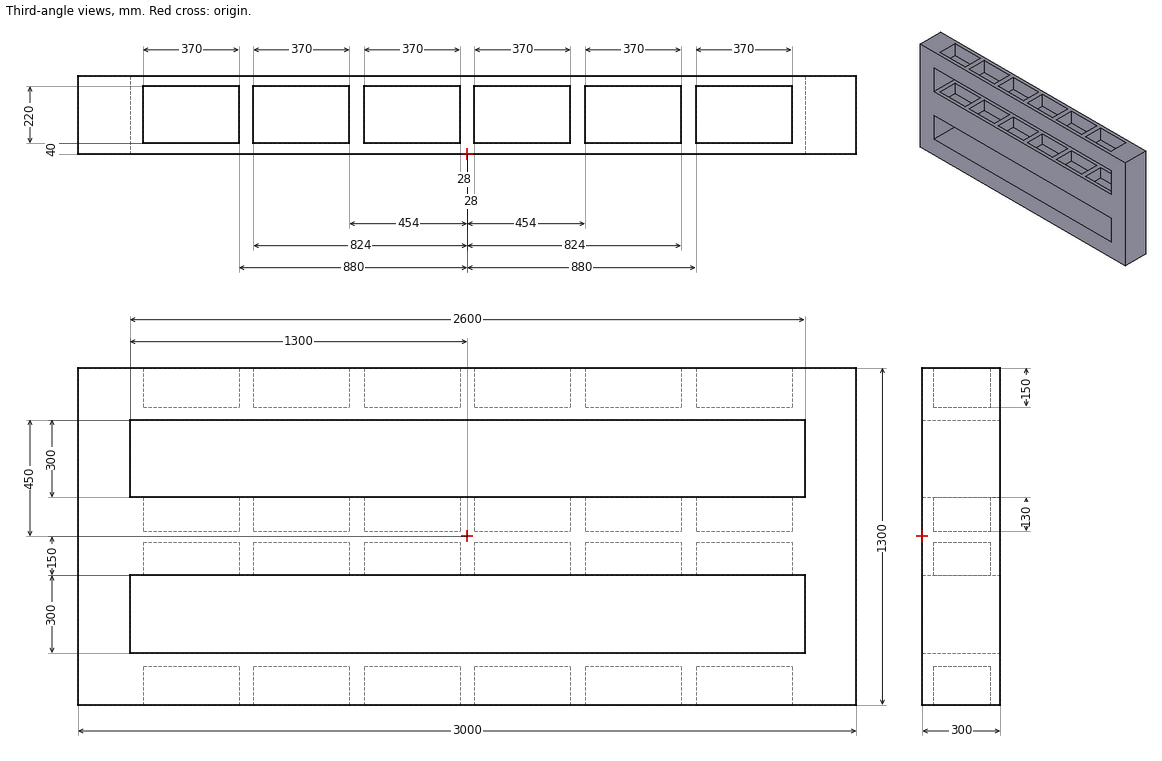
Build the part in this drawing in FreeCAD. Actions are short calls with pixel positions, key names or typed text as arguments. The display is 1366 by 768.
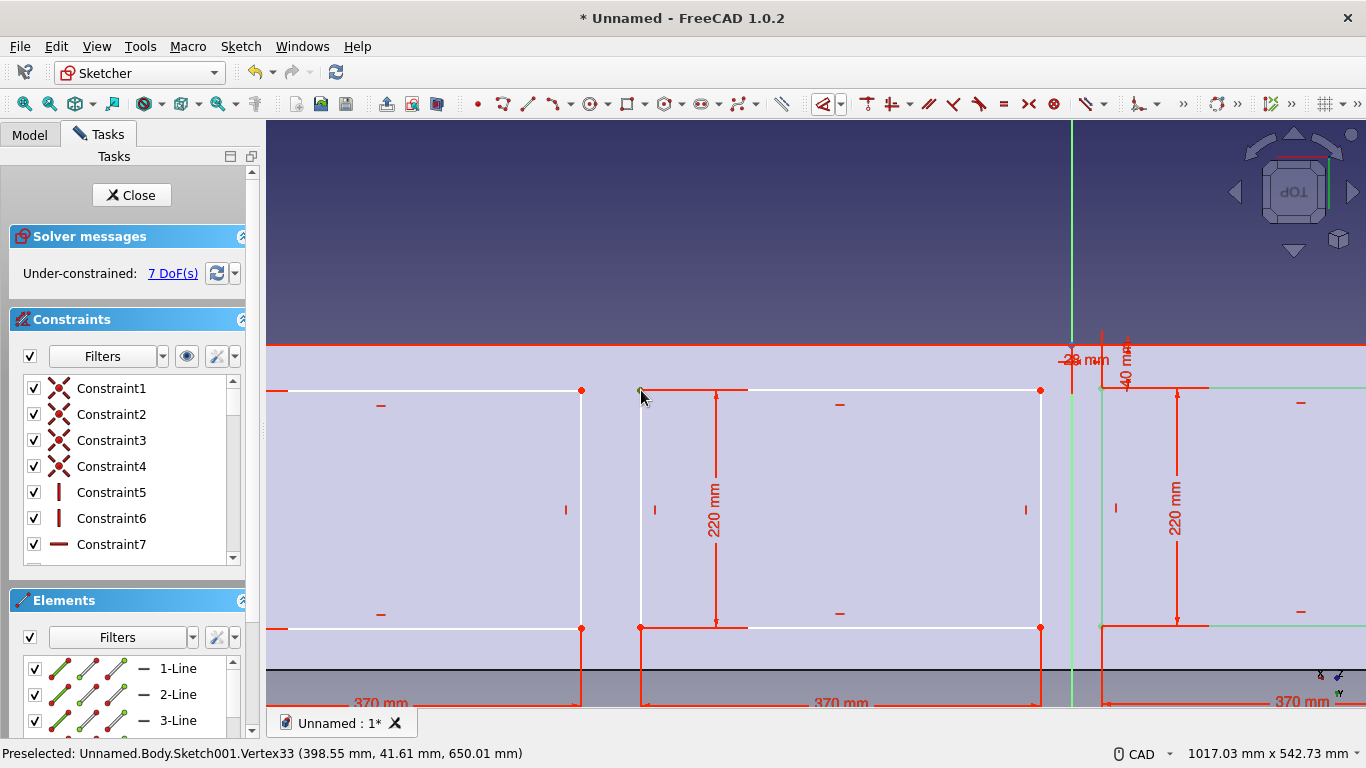
key(i)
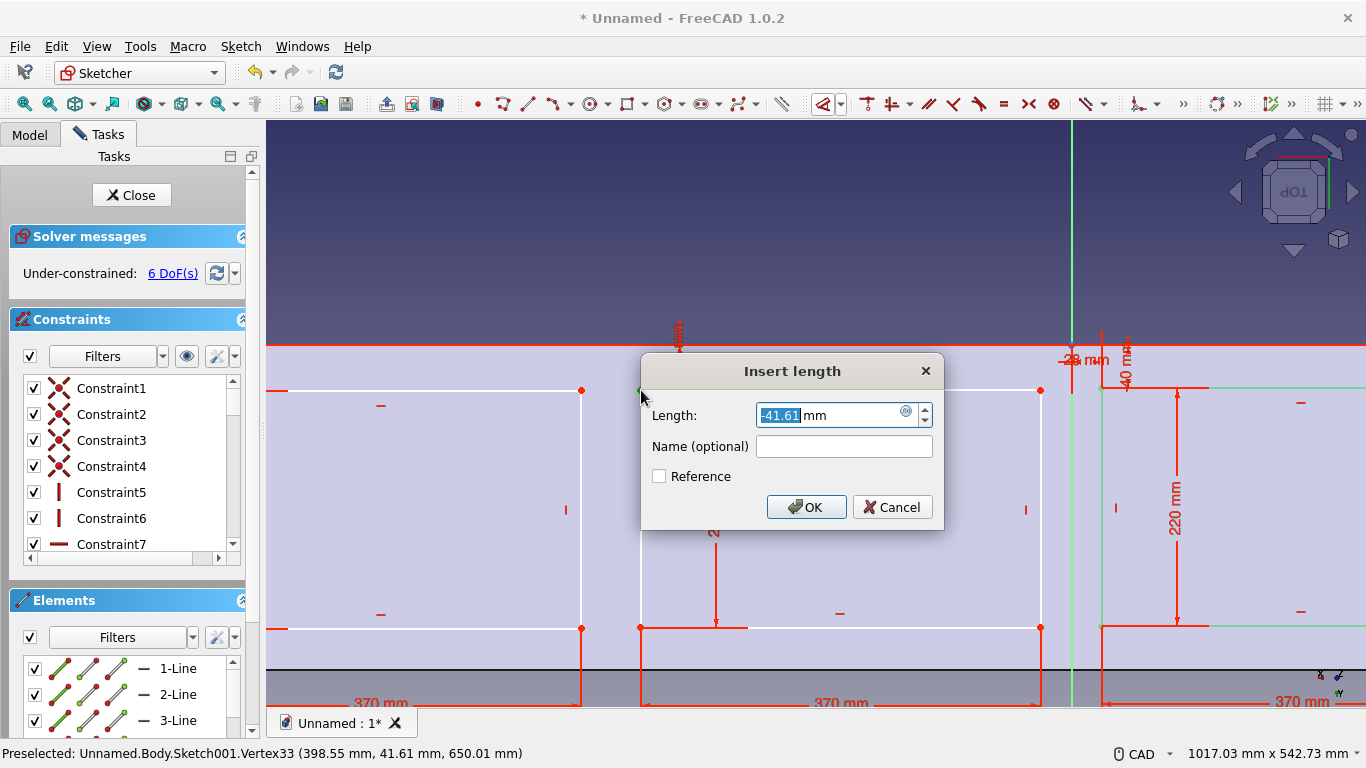
text(-40)
key(Return)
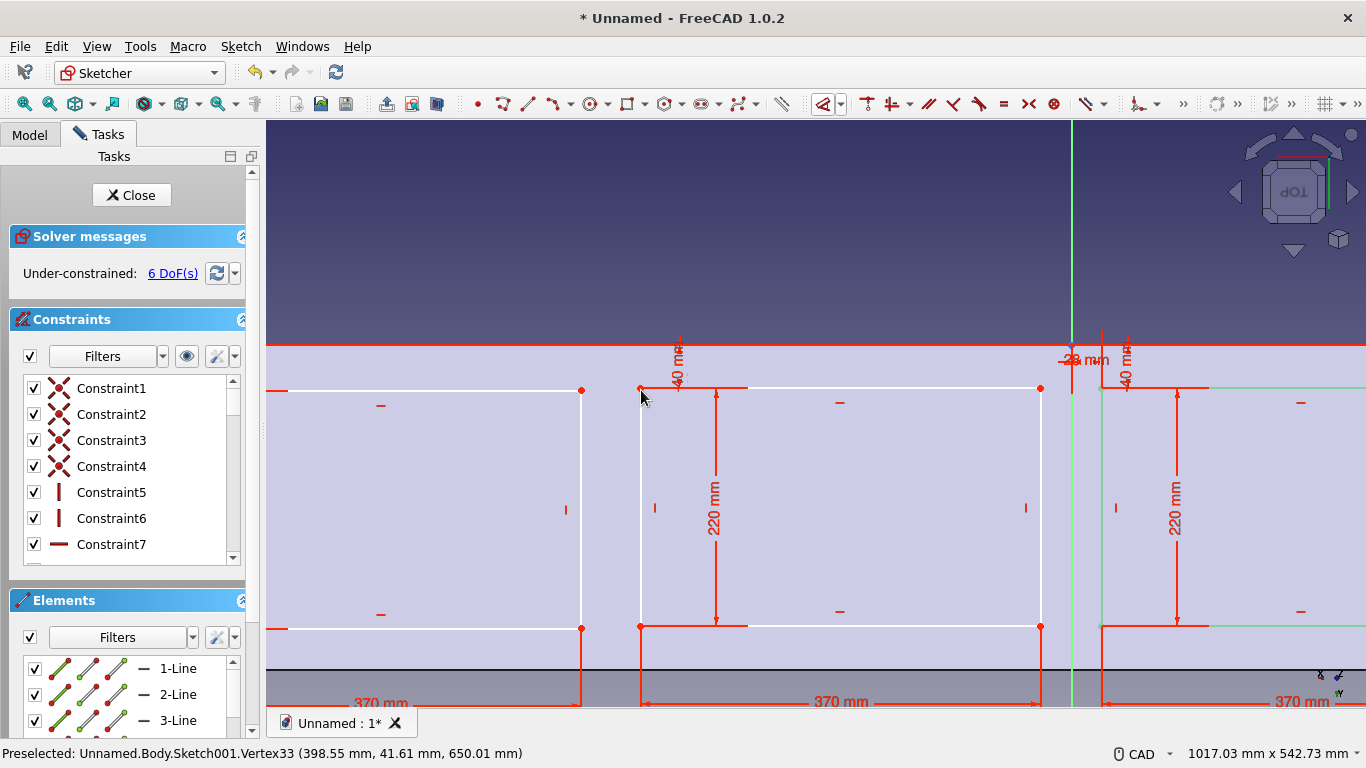
scroll(1041, 626, up, 2)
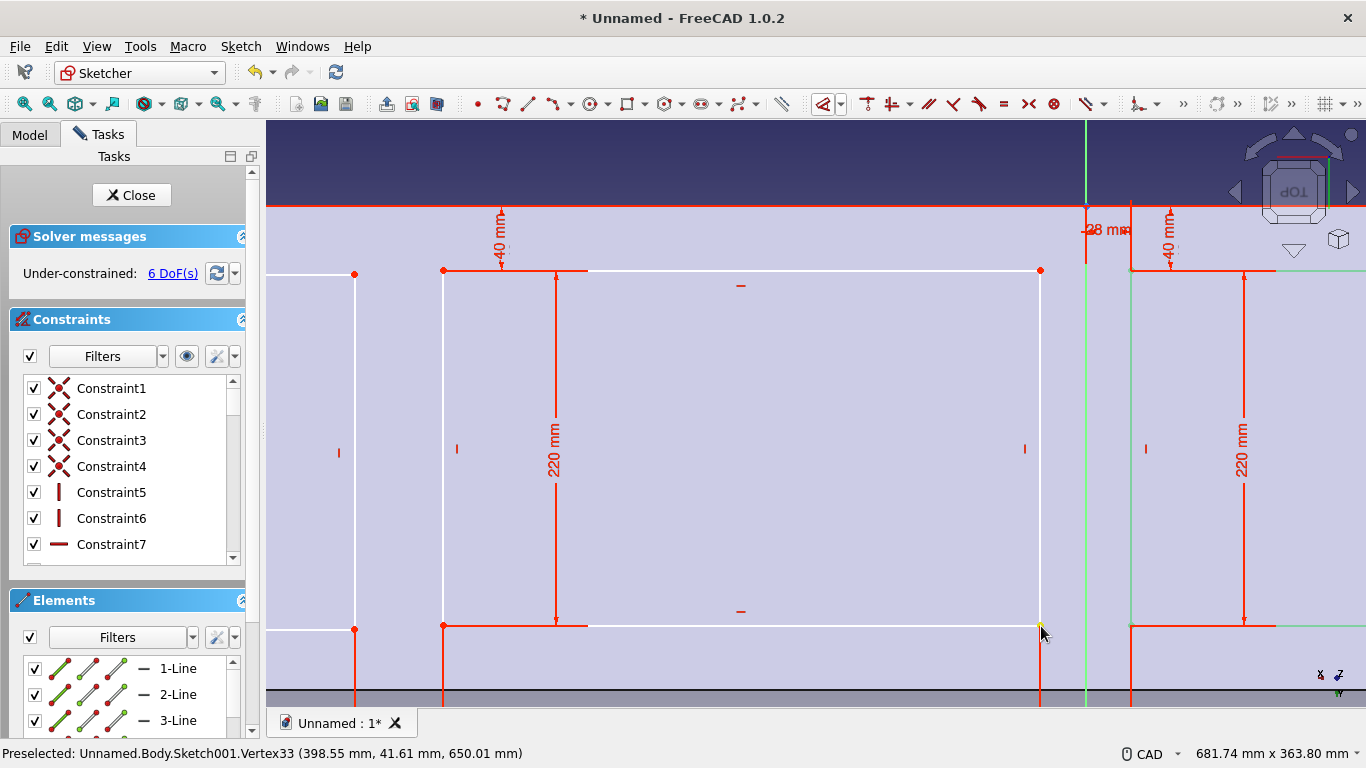
click(1040, 626)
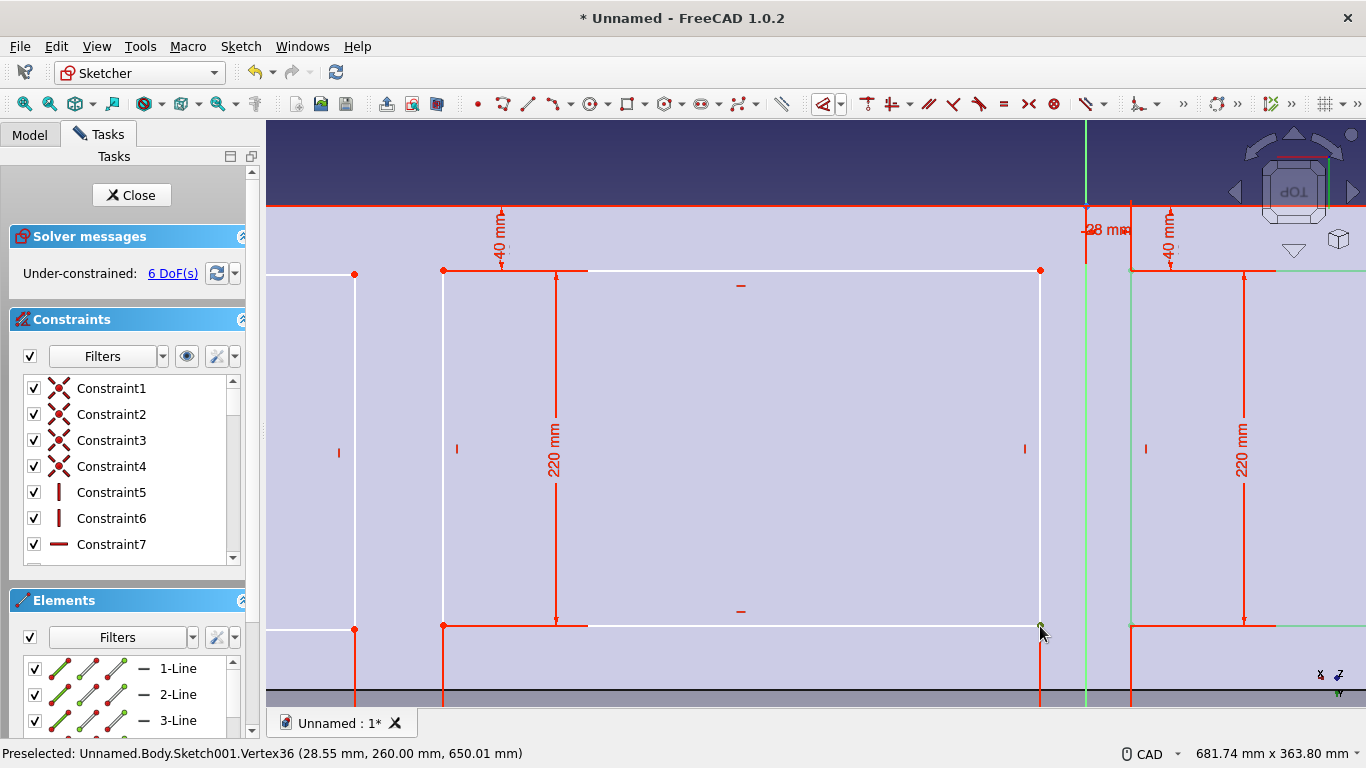
key(l)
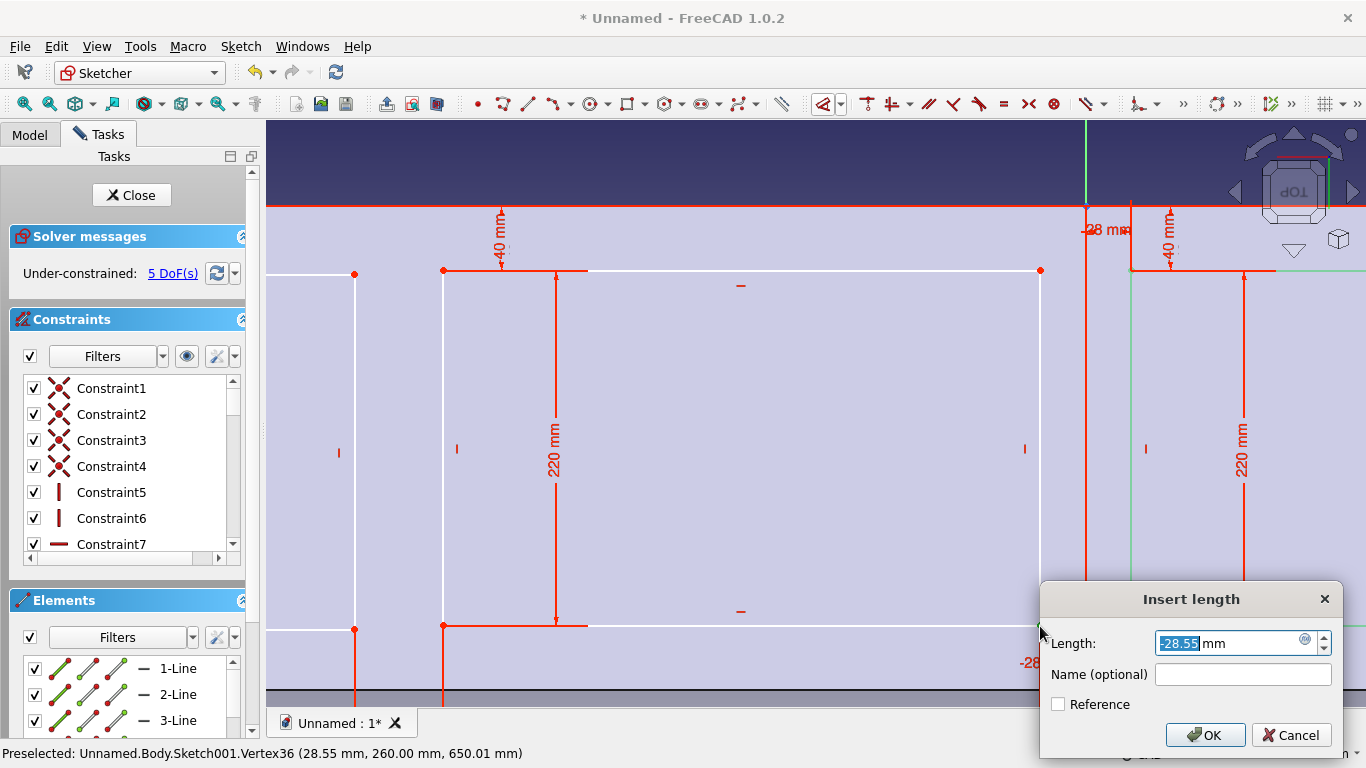
text(-28)
key(Return)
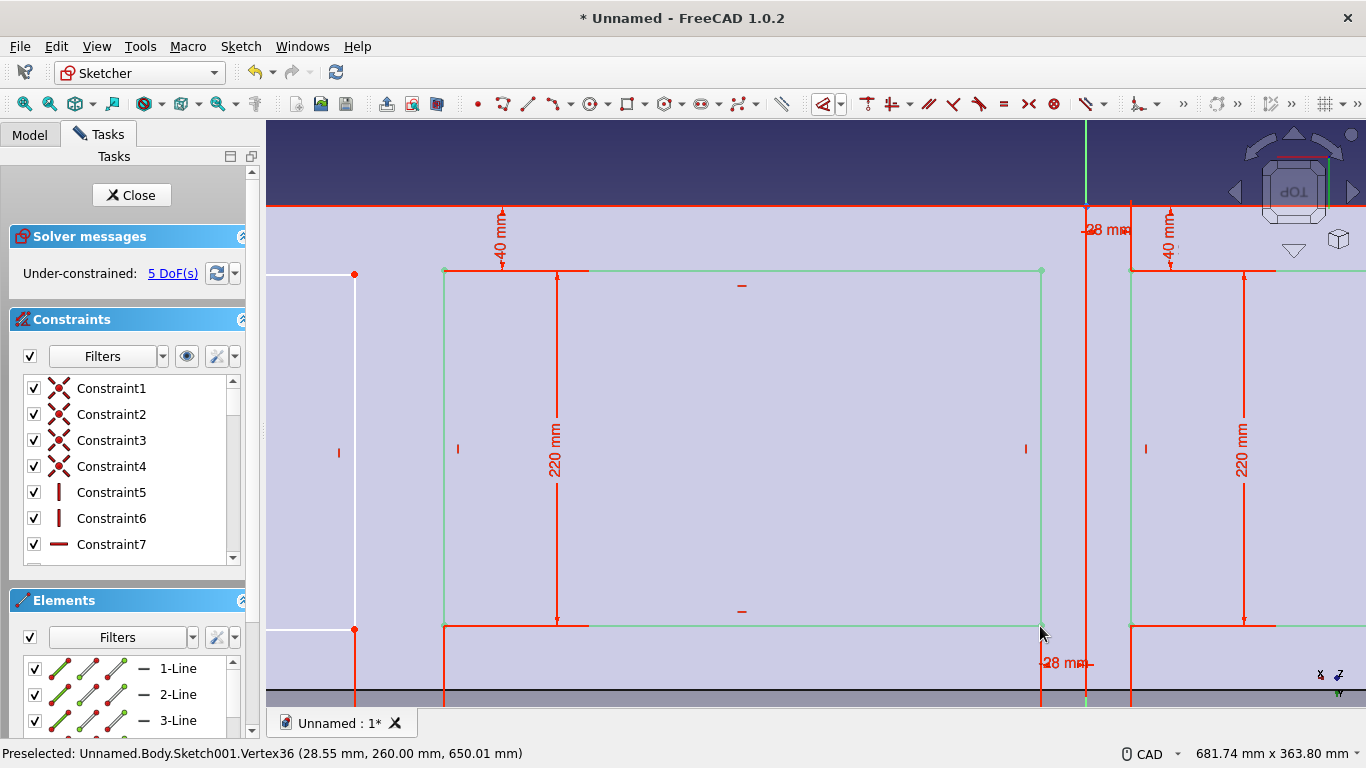
scroll(680, 413, down, 9)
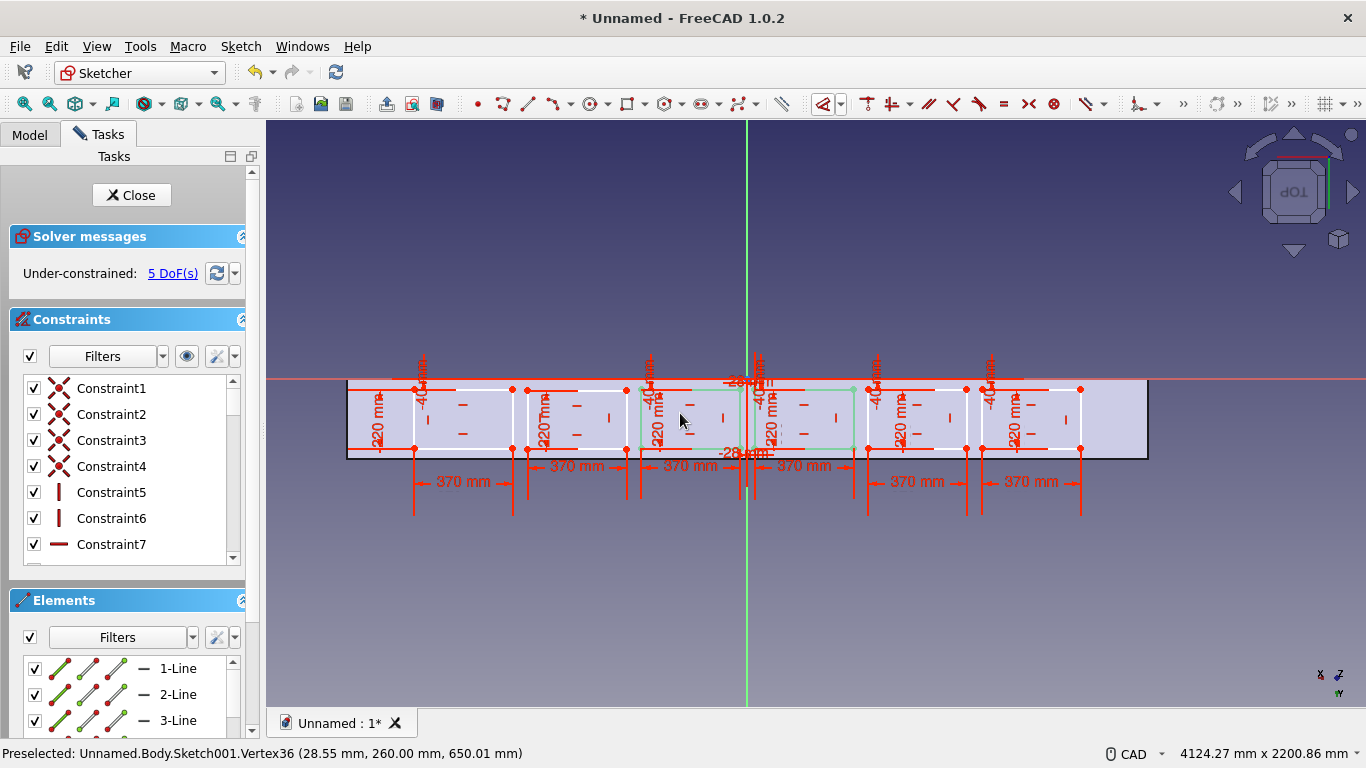
scroll(528, 391, up, 7)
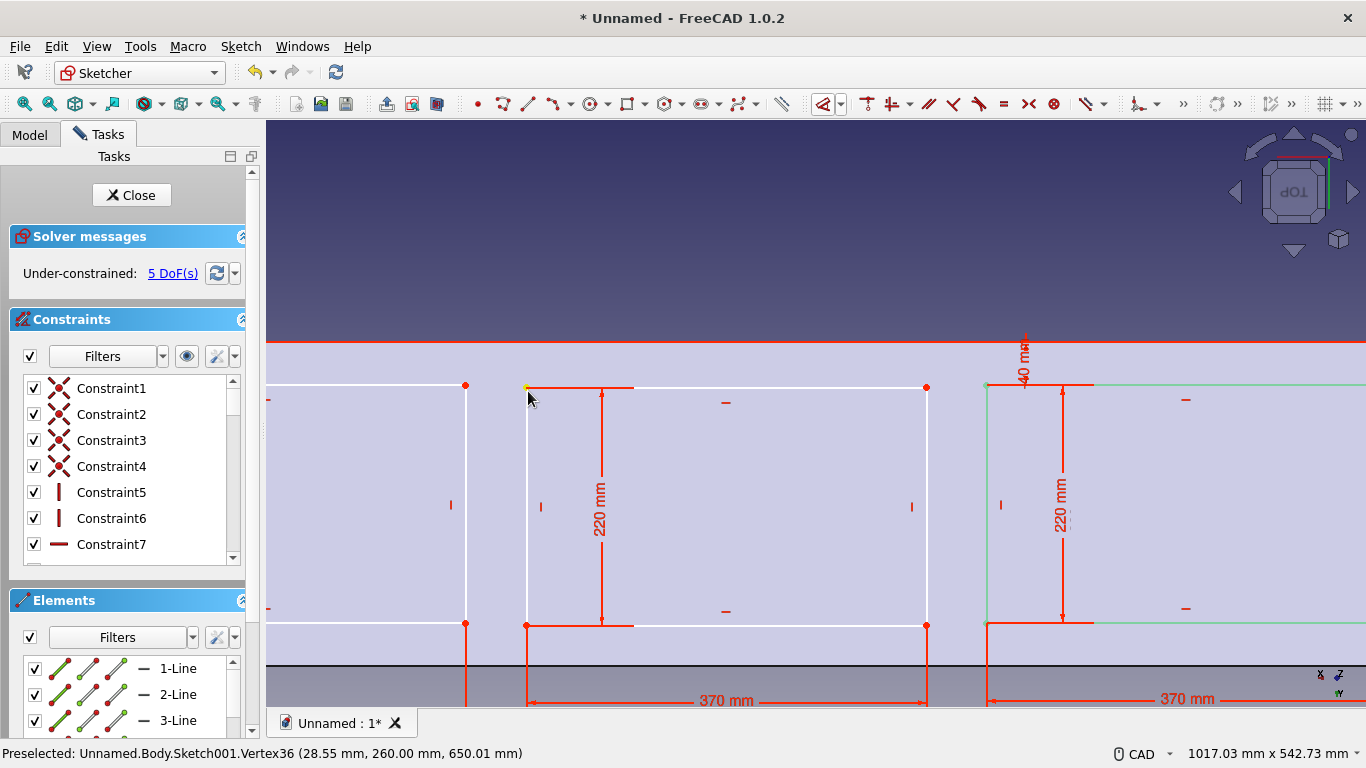
click(527, 388)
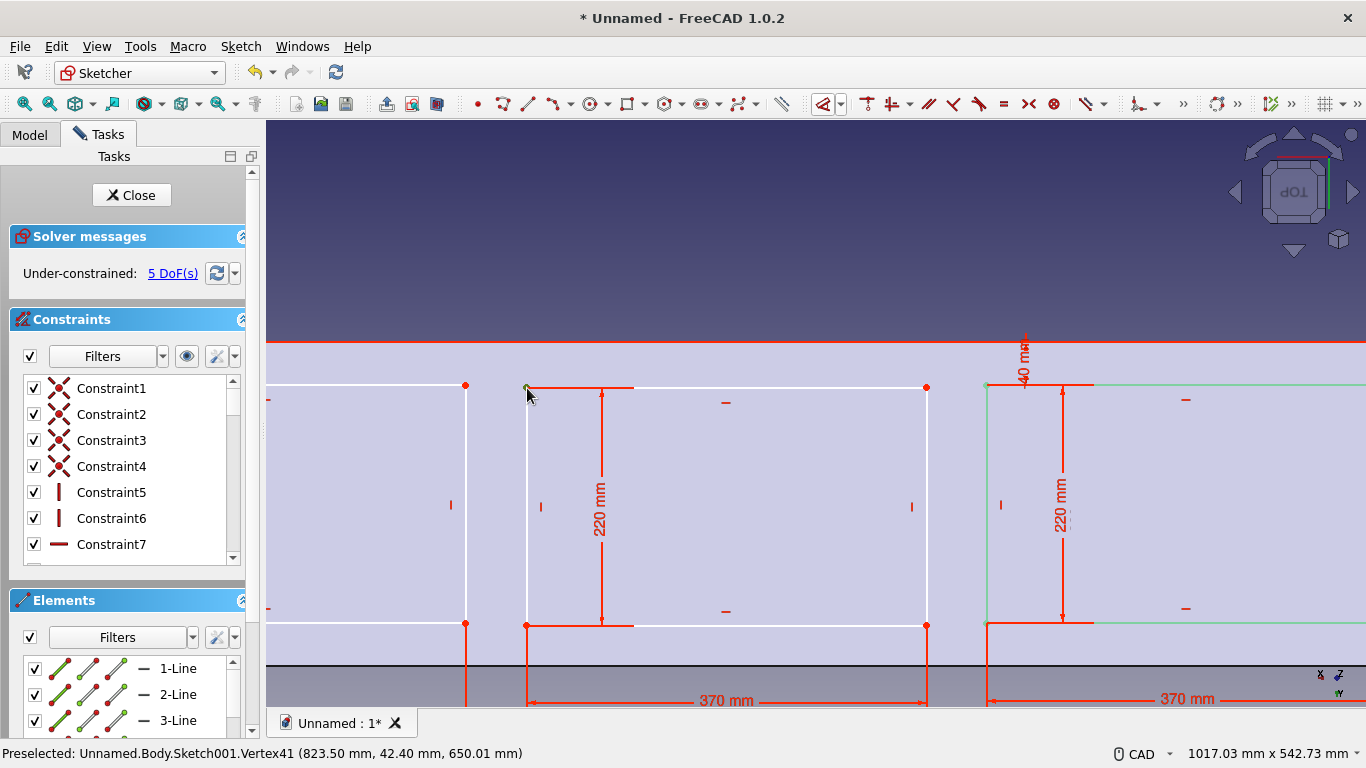
key(i)